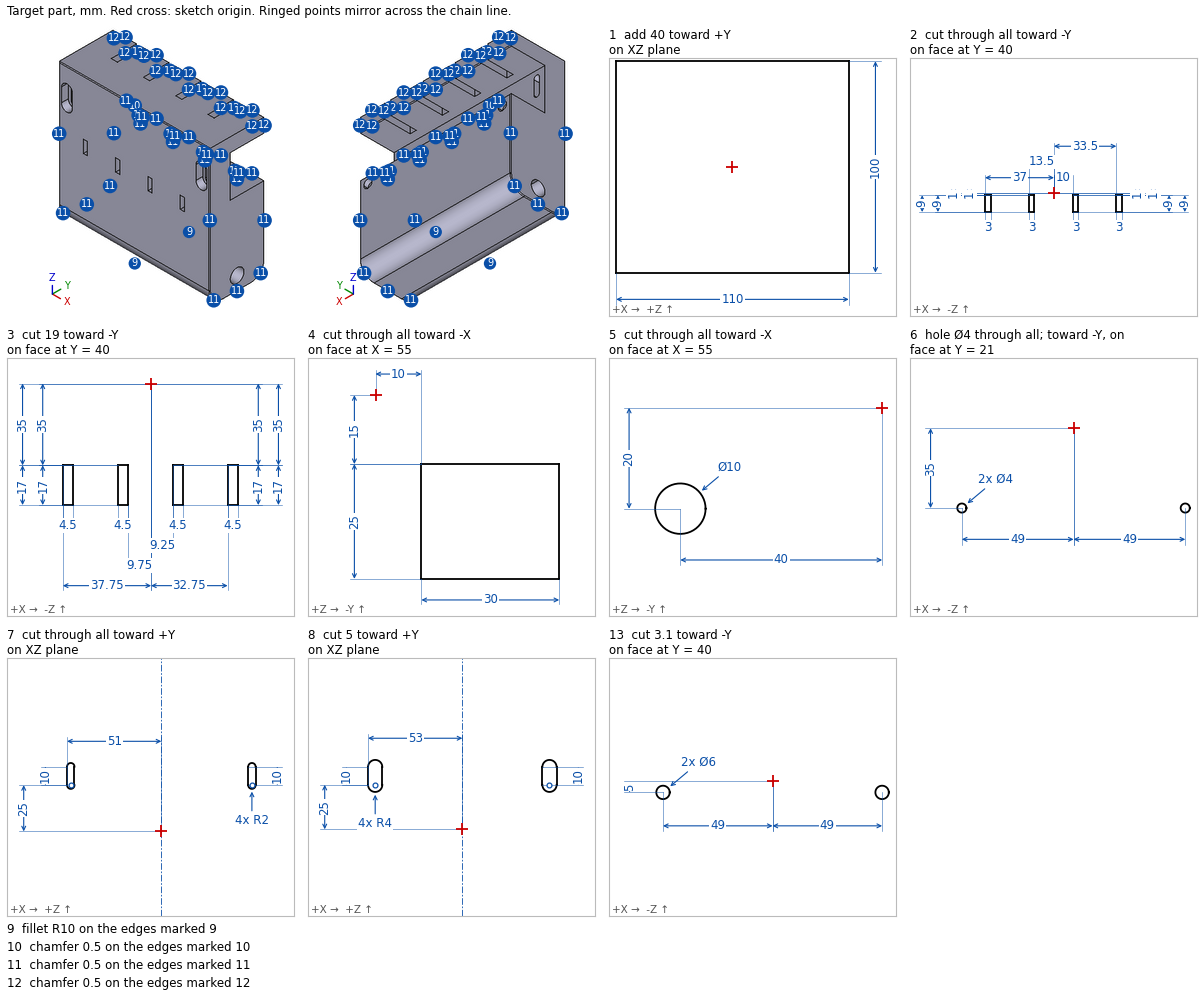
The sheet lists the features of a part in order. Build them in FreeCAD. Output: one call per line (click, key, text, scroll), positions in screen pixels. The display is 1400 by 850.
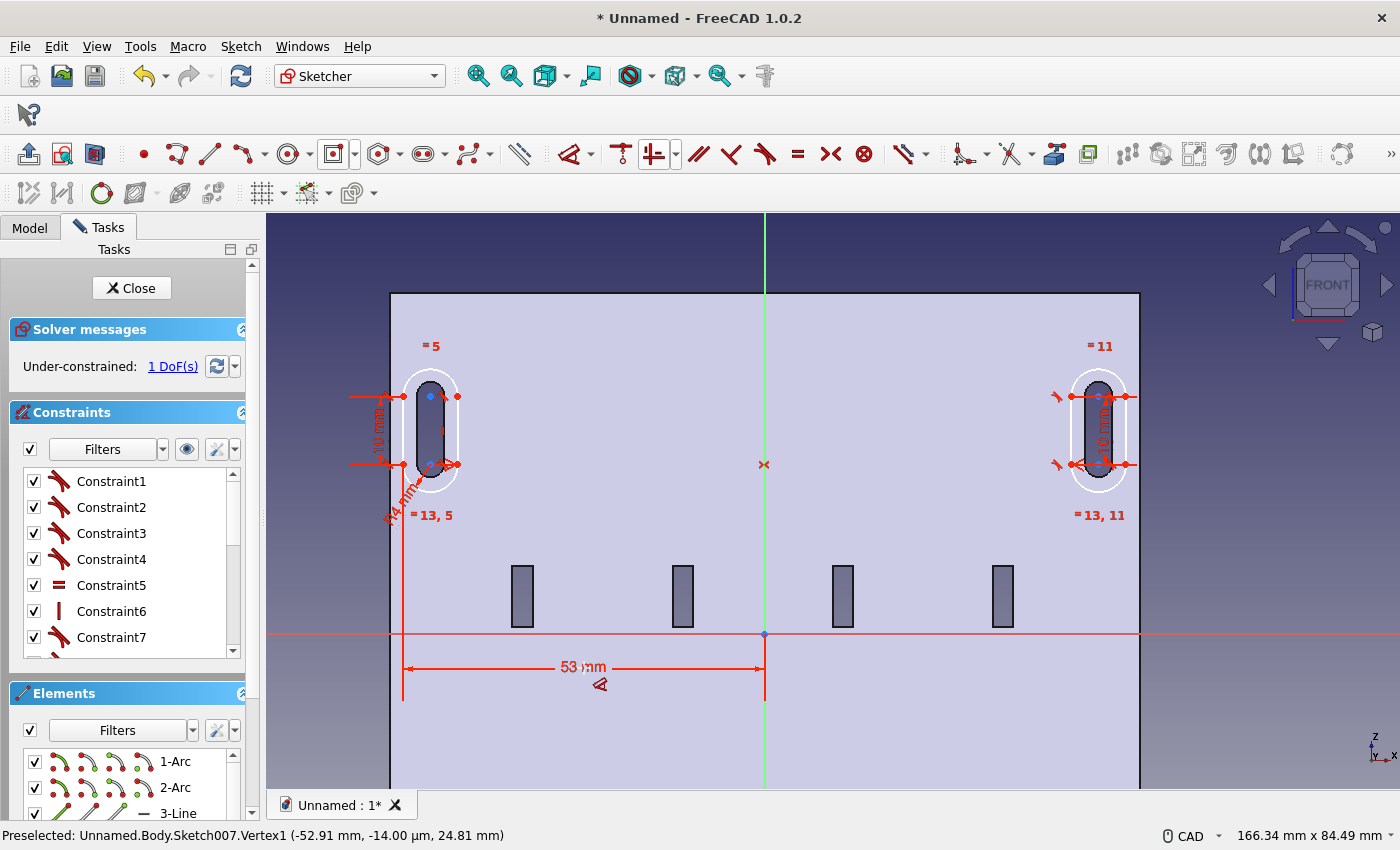
click(403, 465)
click(369, 549)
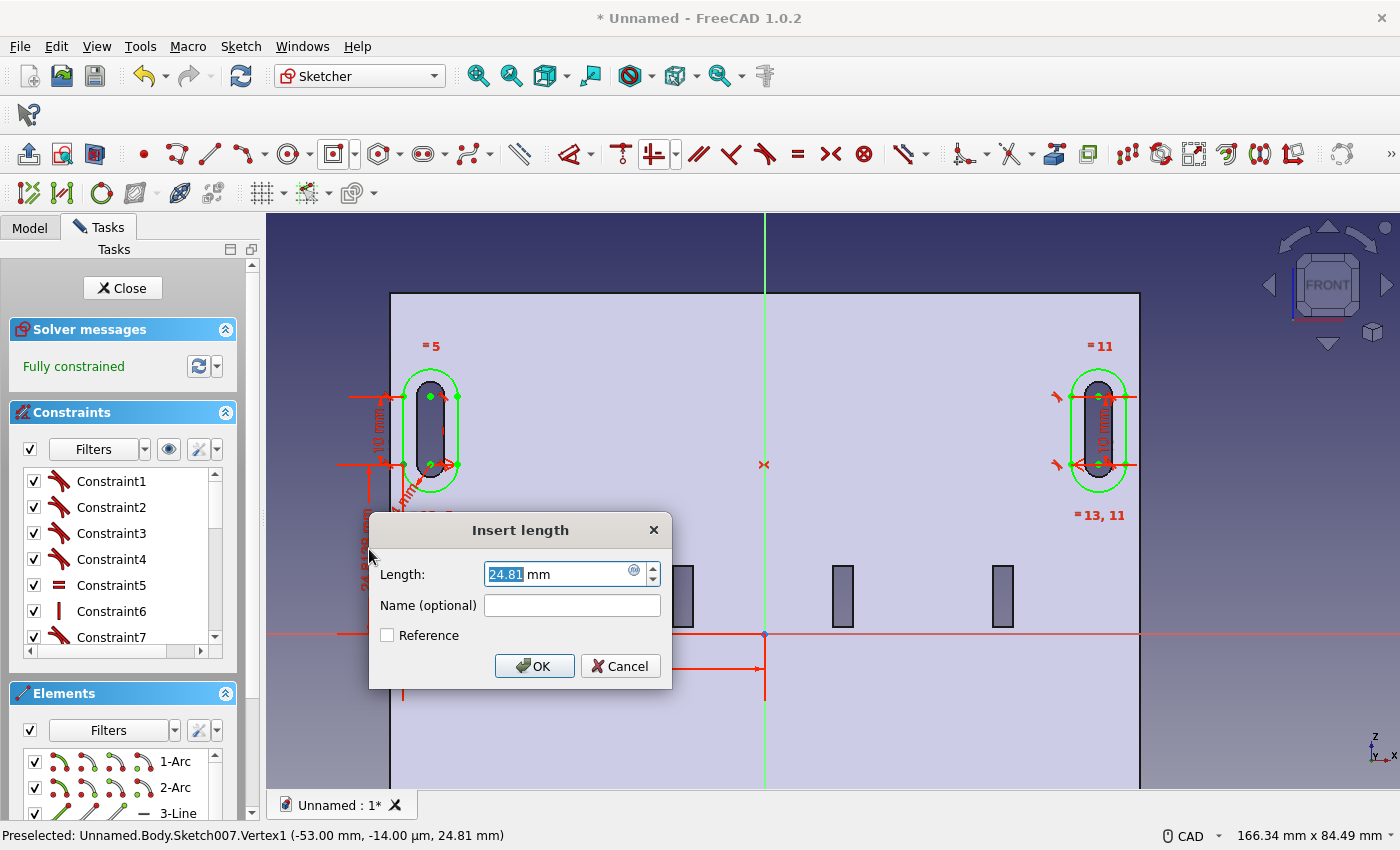
text(25)
key(Return)
key(Escape)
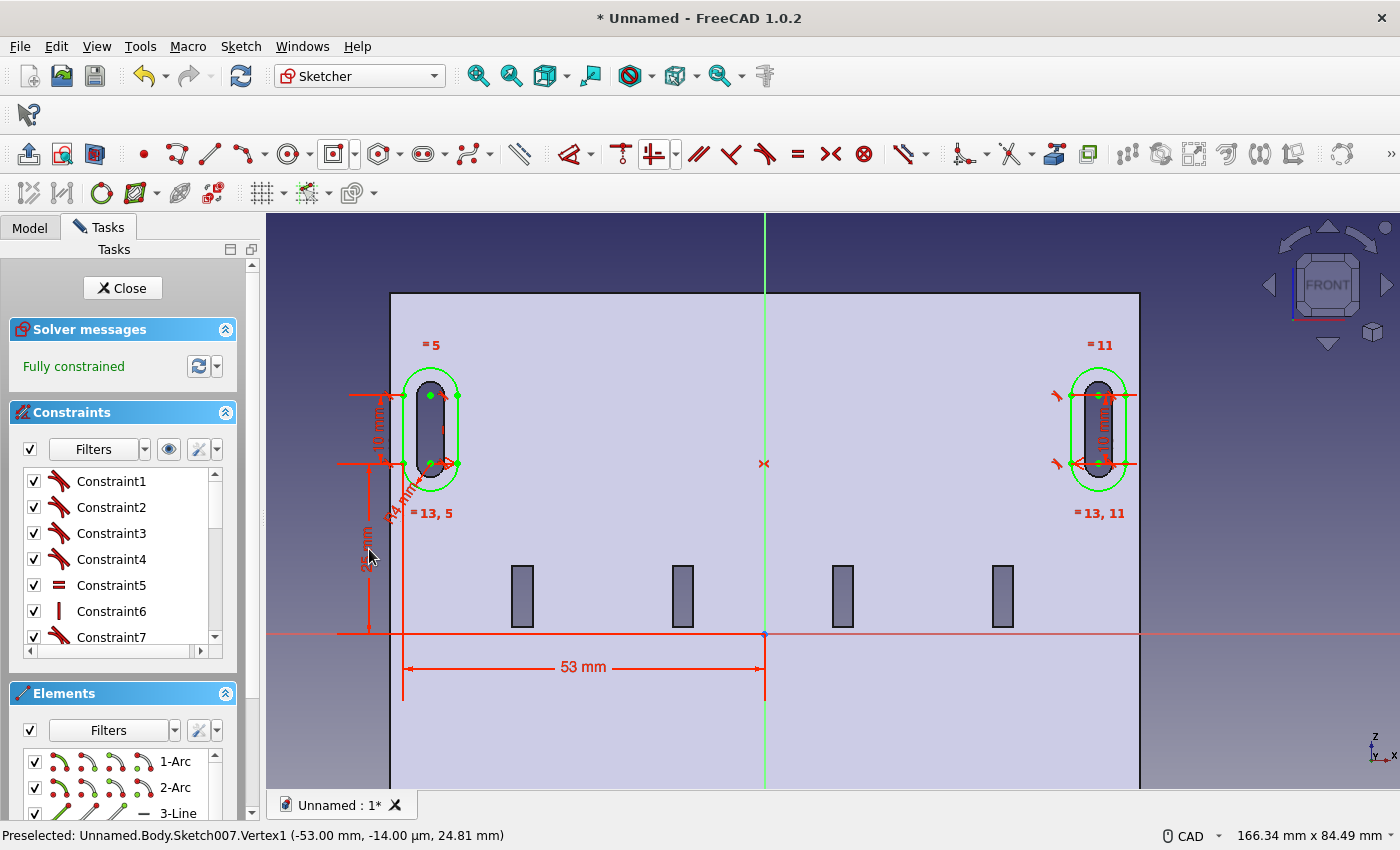
click(123, 288)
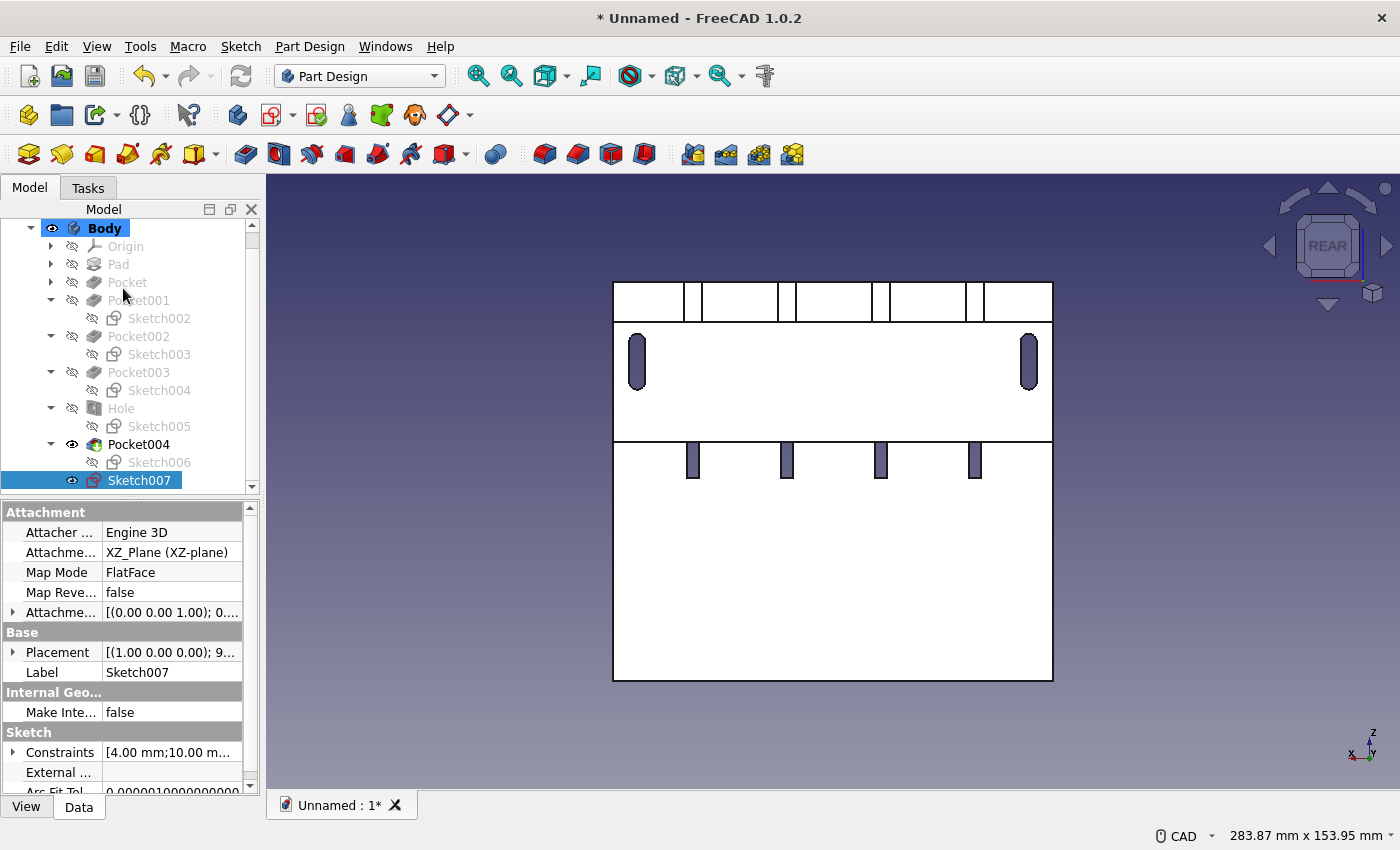
click(246, 154)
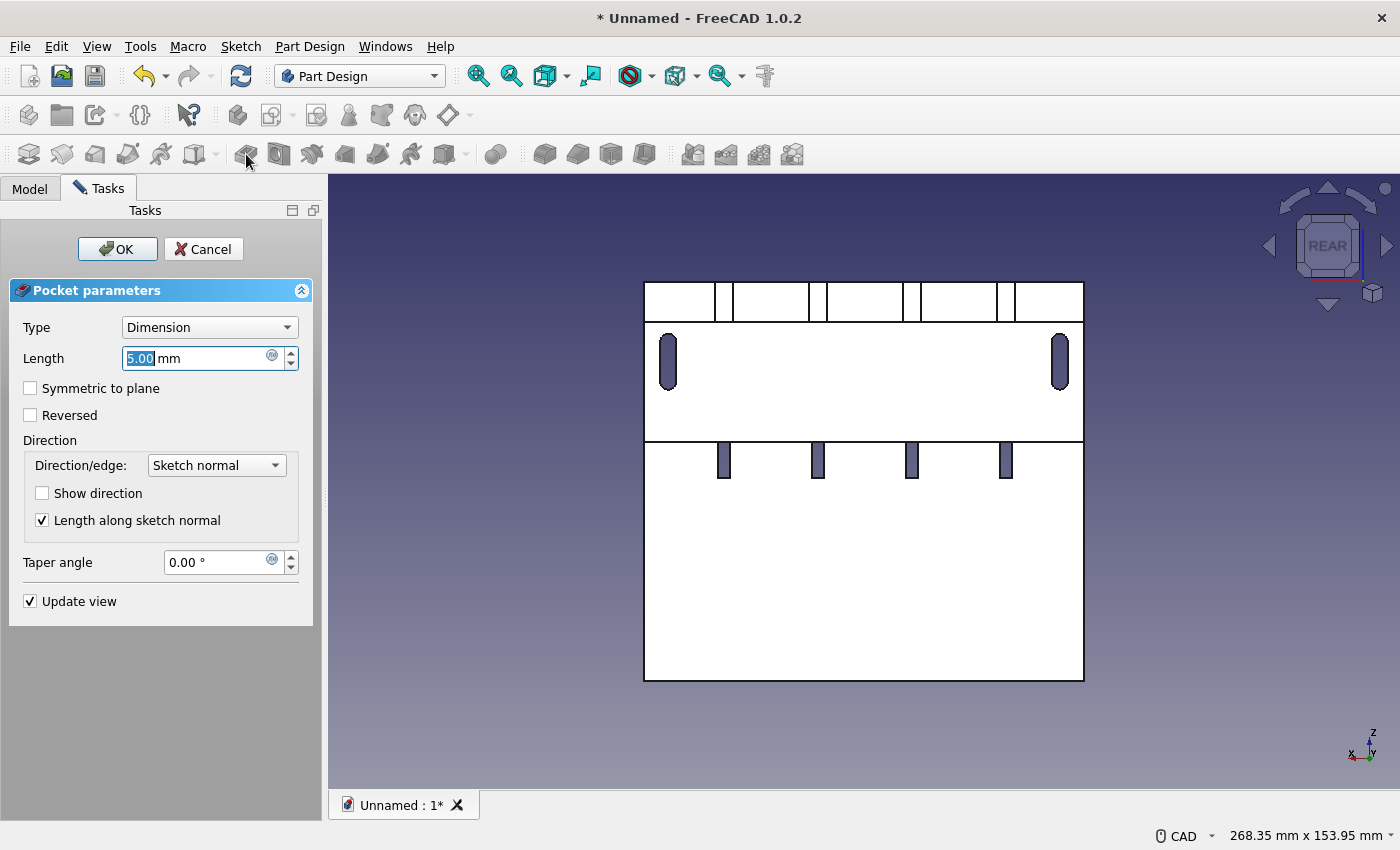
text(5)
key(Tab)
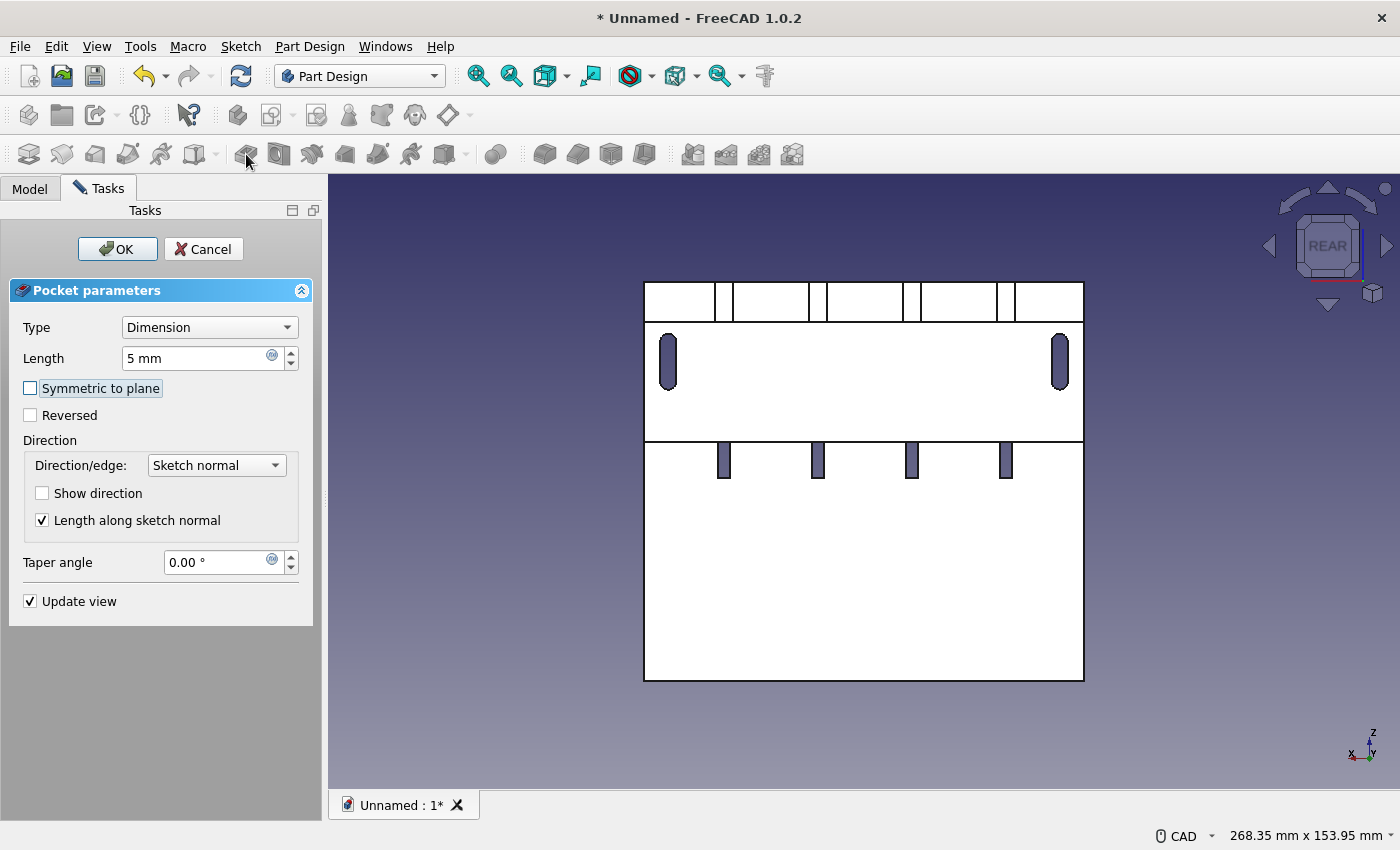
click(118, 249)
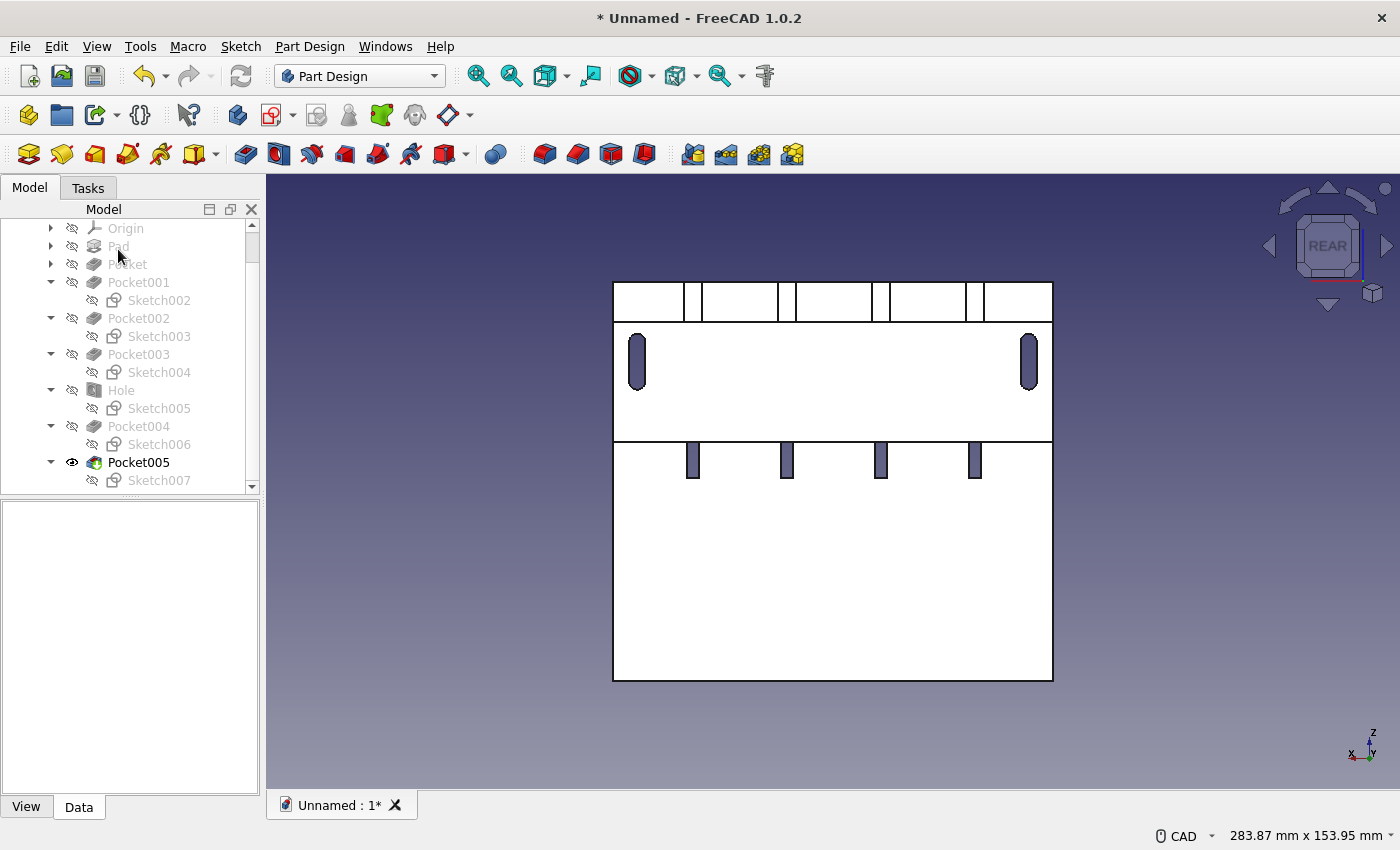
click(833, 680)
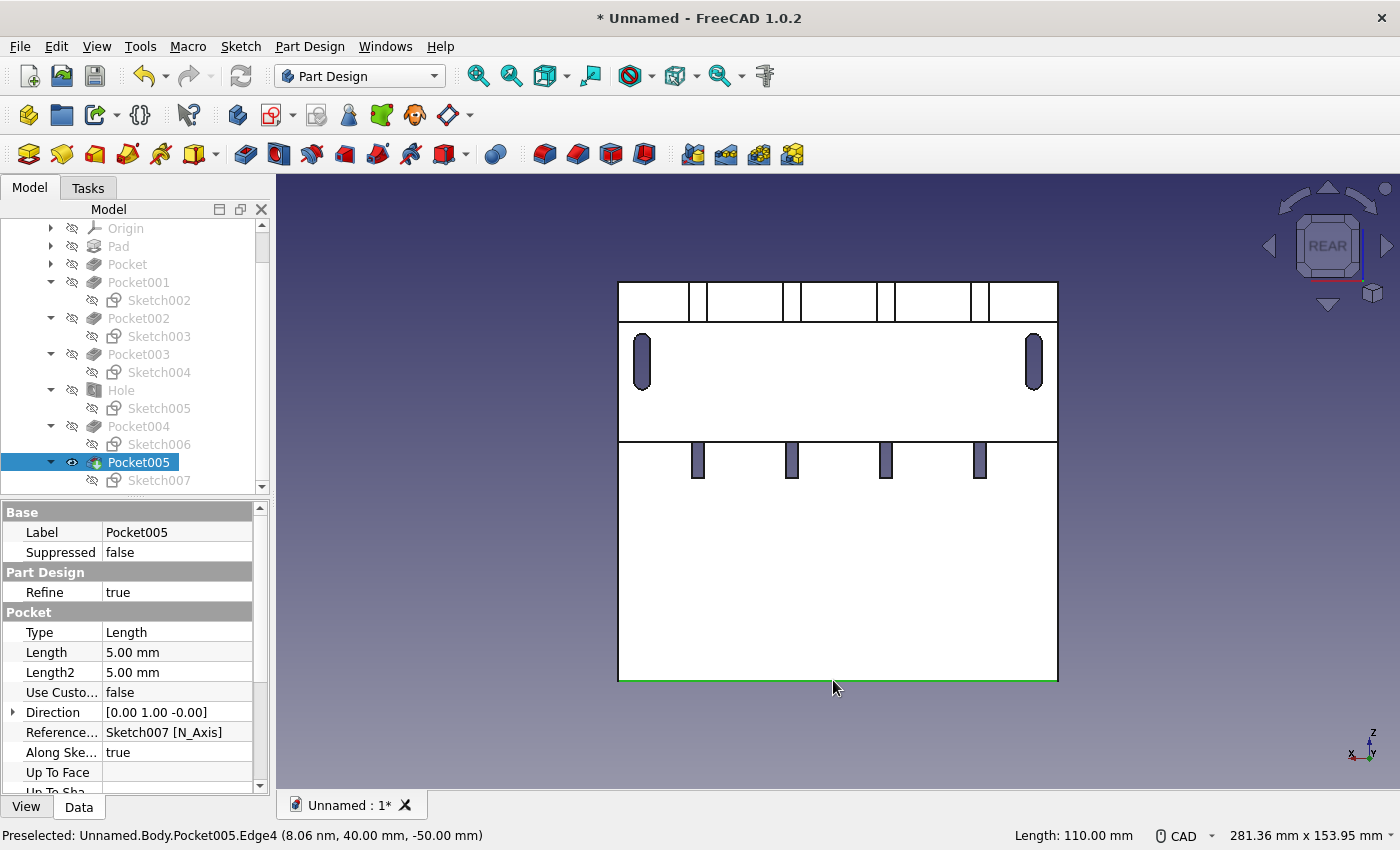
key(0)